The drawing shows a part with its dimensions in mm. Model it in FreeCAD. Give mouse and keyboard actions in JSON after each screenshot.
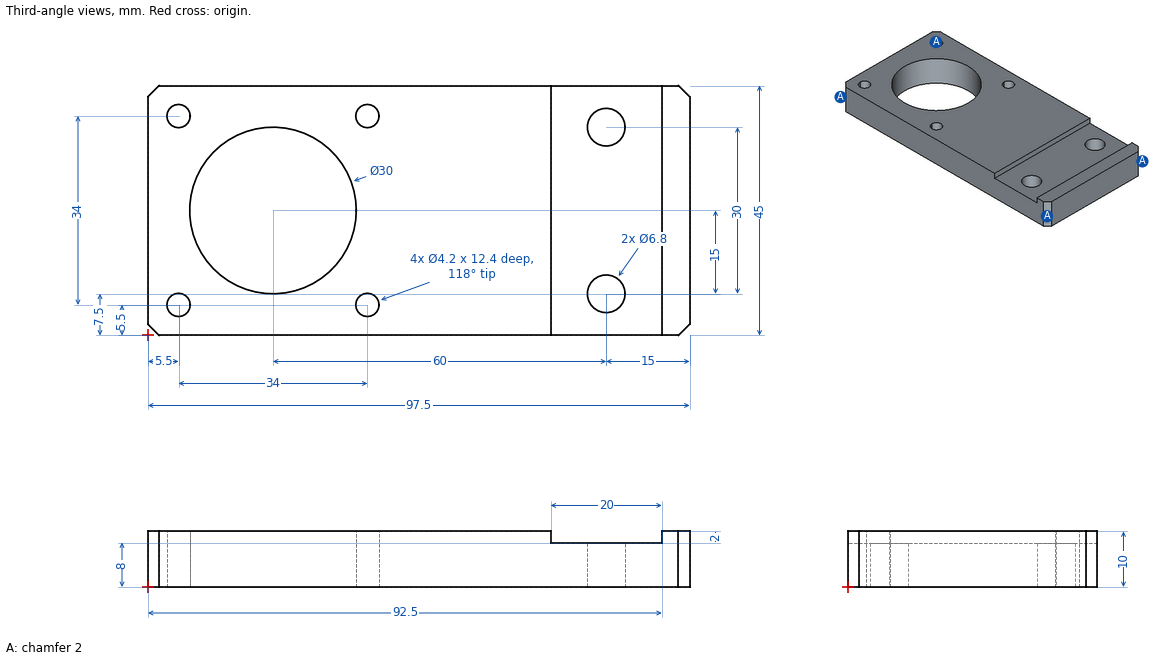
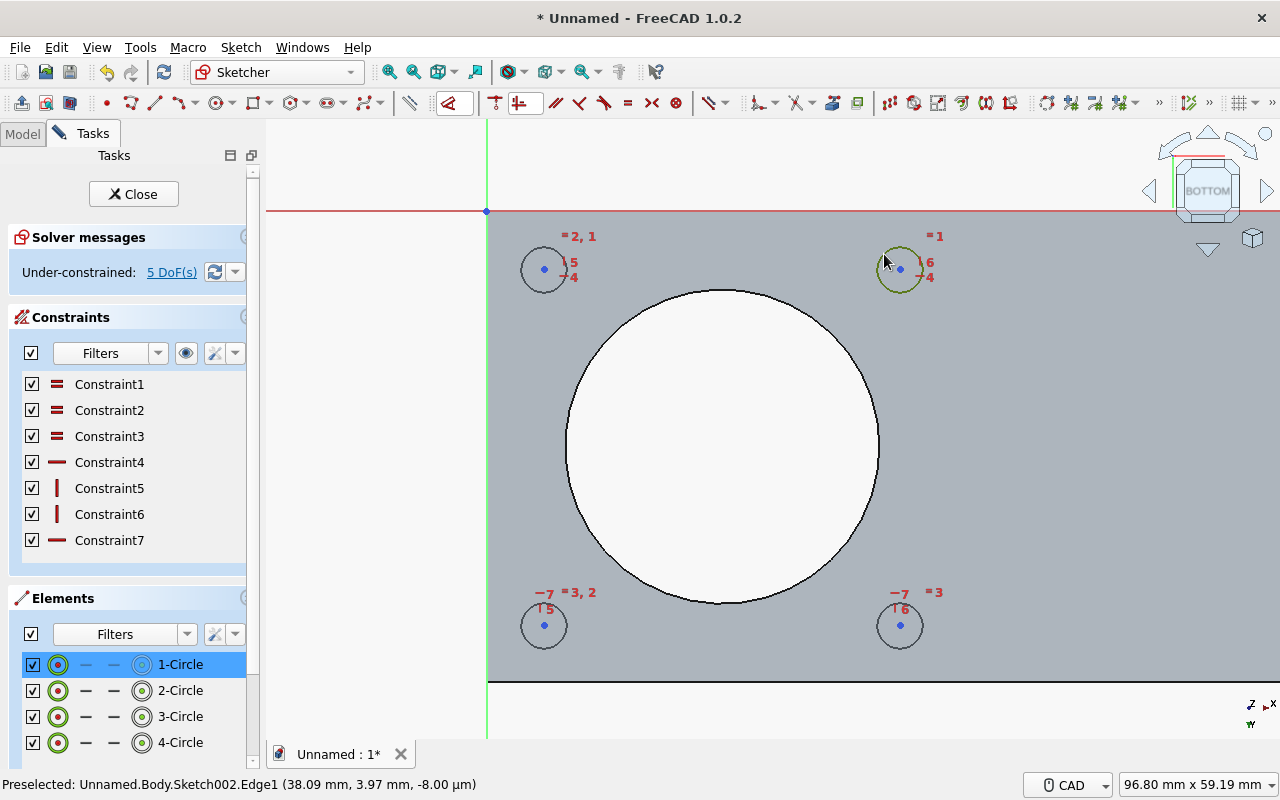
{"action": "left_click", "coordinate": [468, 104]}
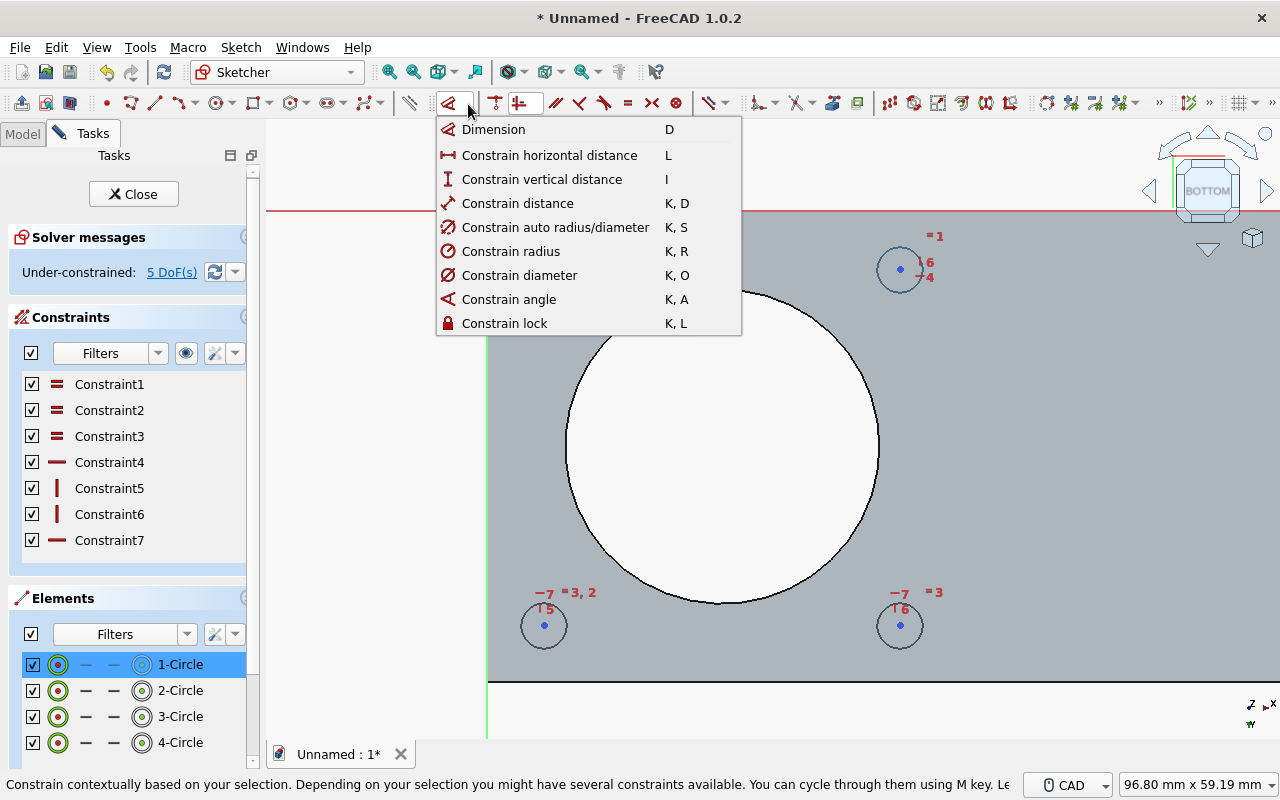
{"action": "left_click", "coordinate": [589, 275]}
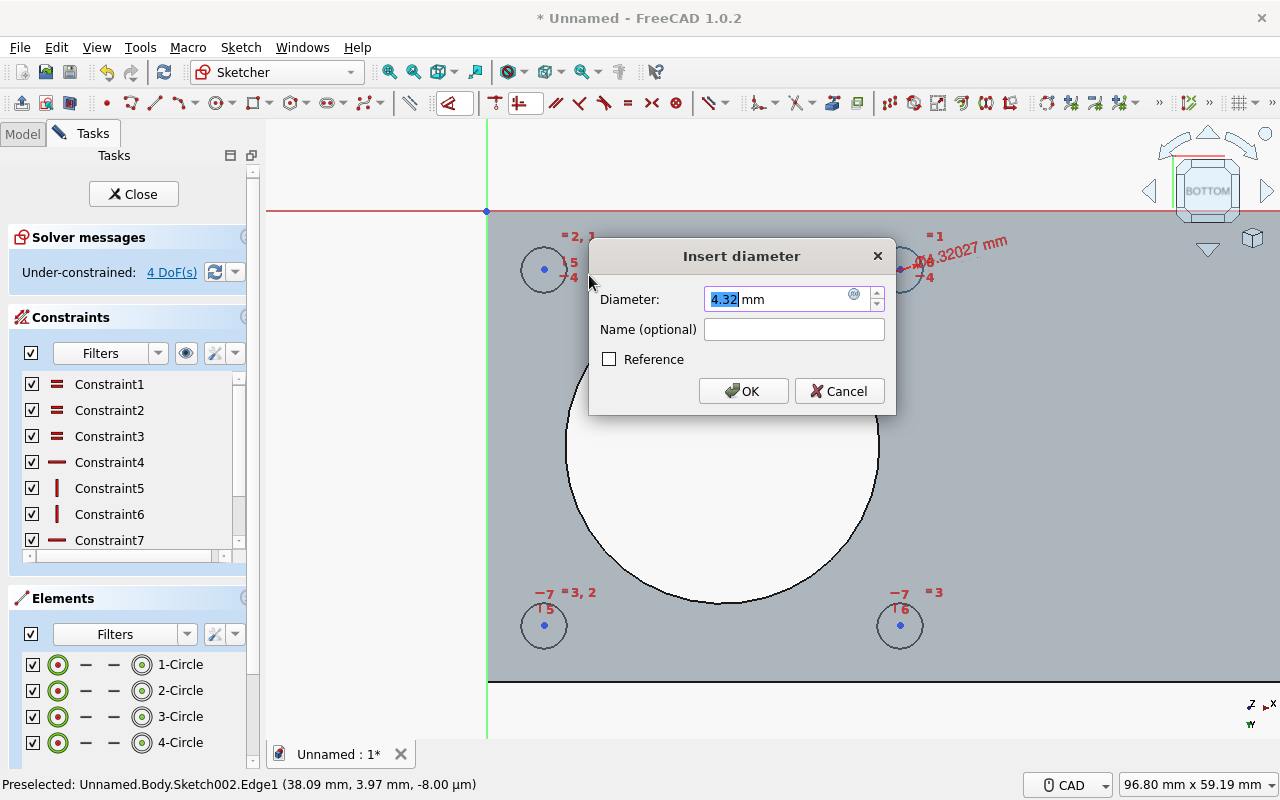
{"action": "type", "text": "4.2"}
{"action": "key", "text": "Return"}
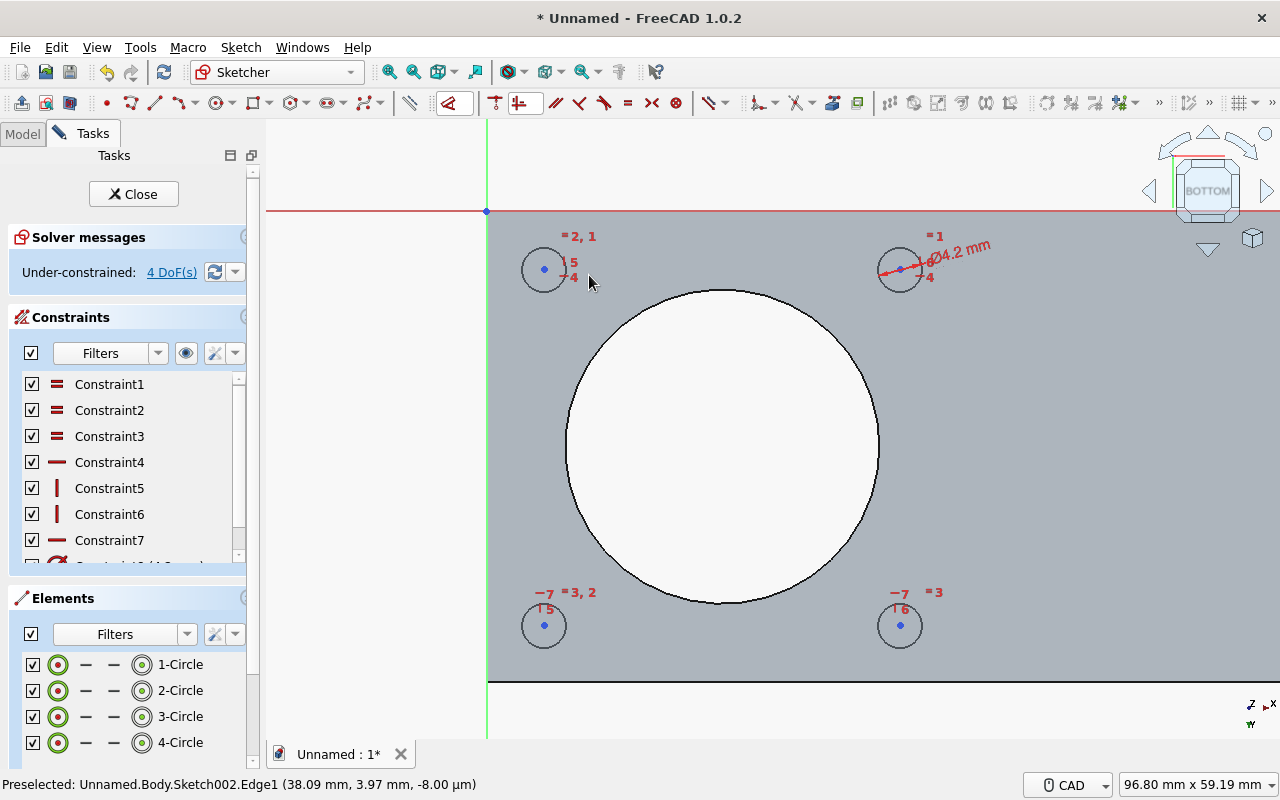
{"action": "left_click", "coordinate": [900, 270]}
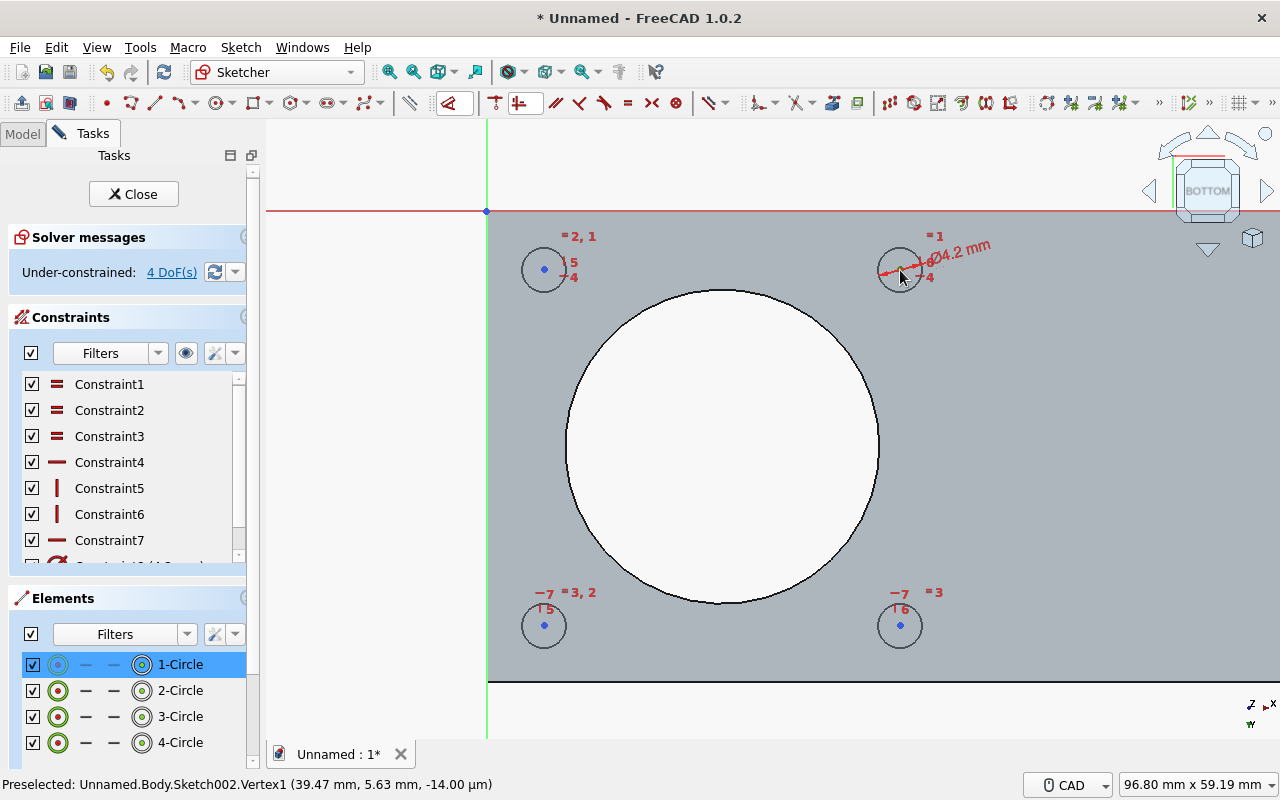
{"action": "key", "text": "i"}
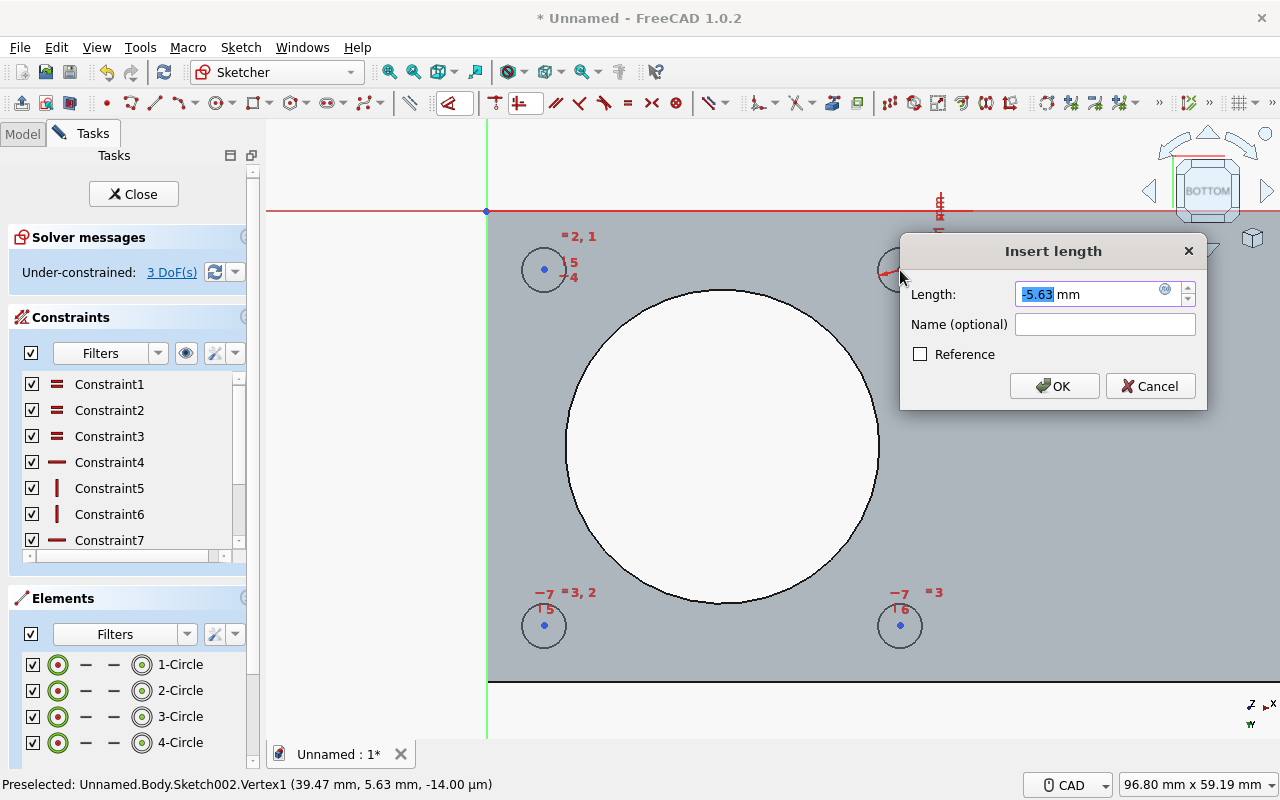
{"action": "type", "text": "-5.5"}
{"action": "key", "text": "Return"}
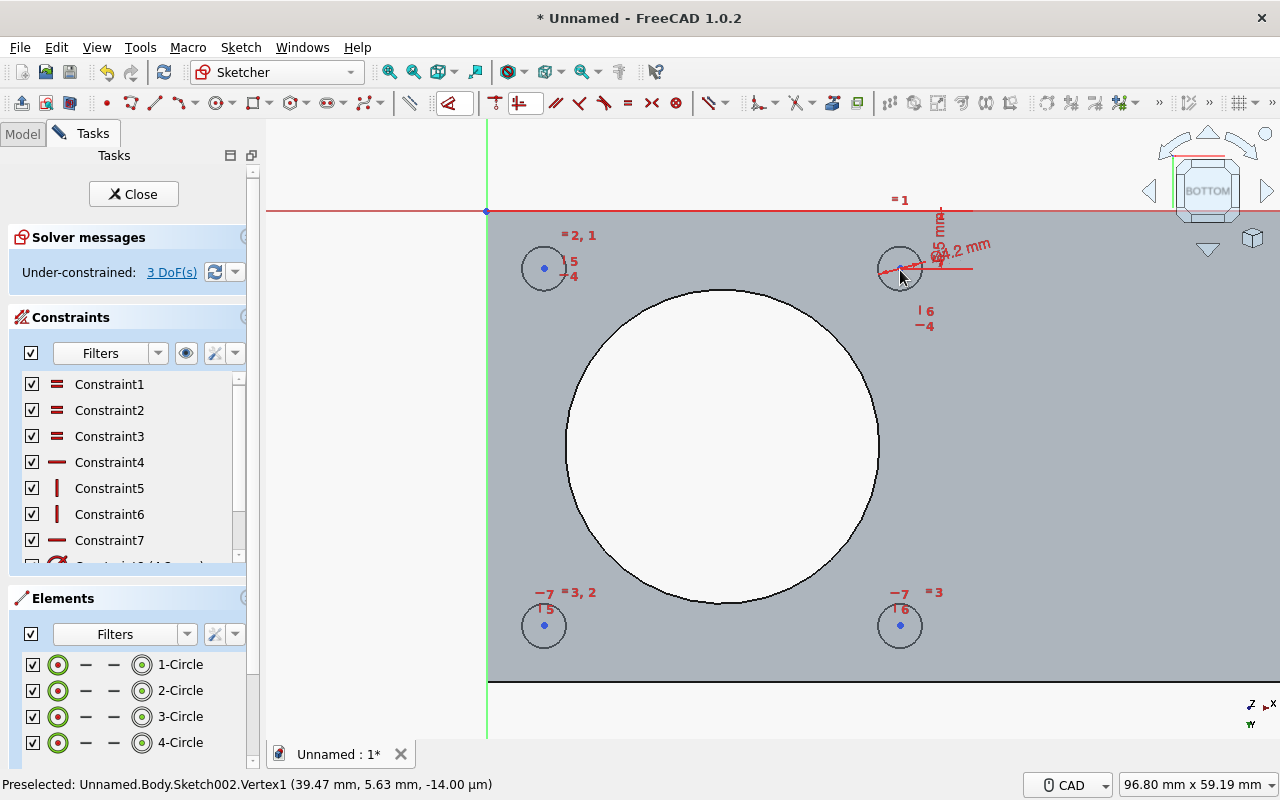
{"action": "left_click", "coordinate": [544, 269]}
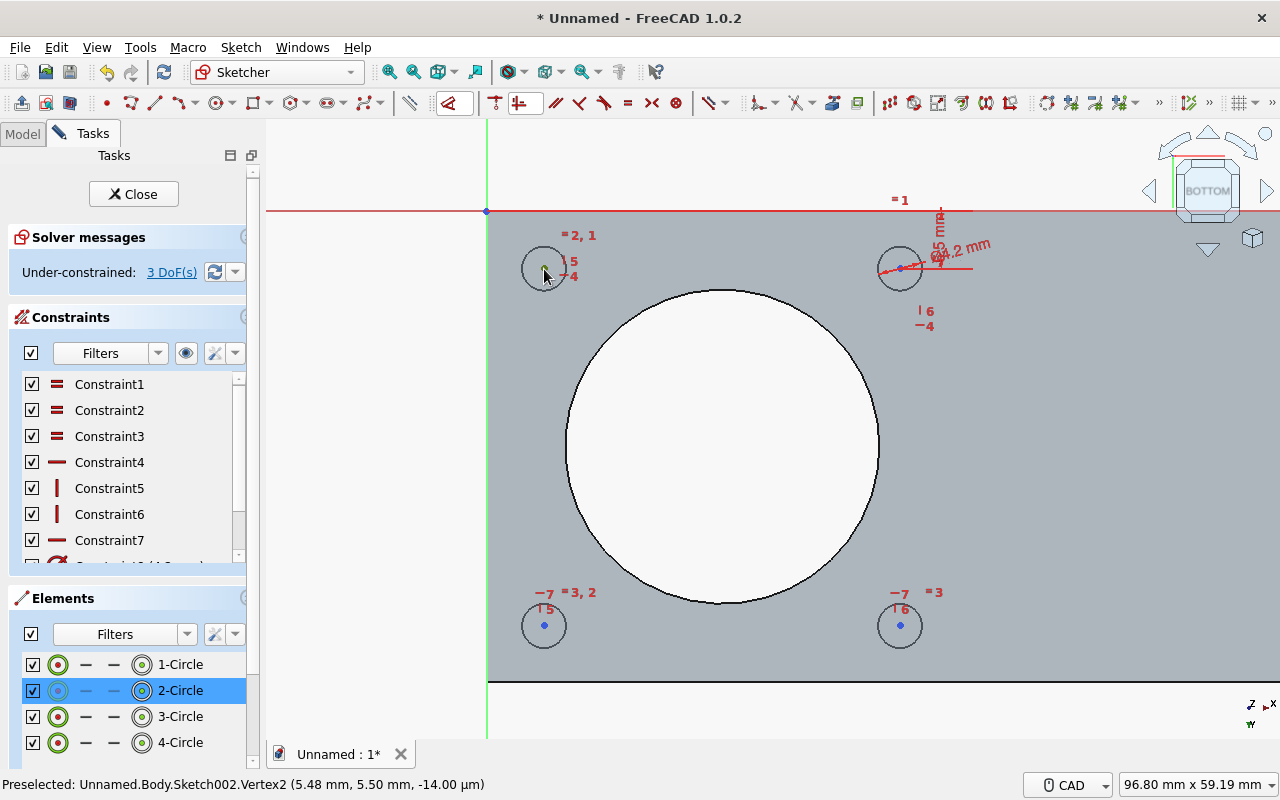
{"action": "key", "text": "l"}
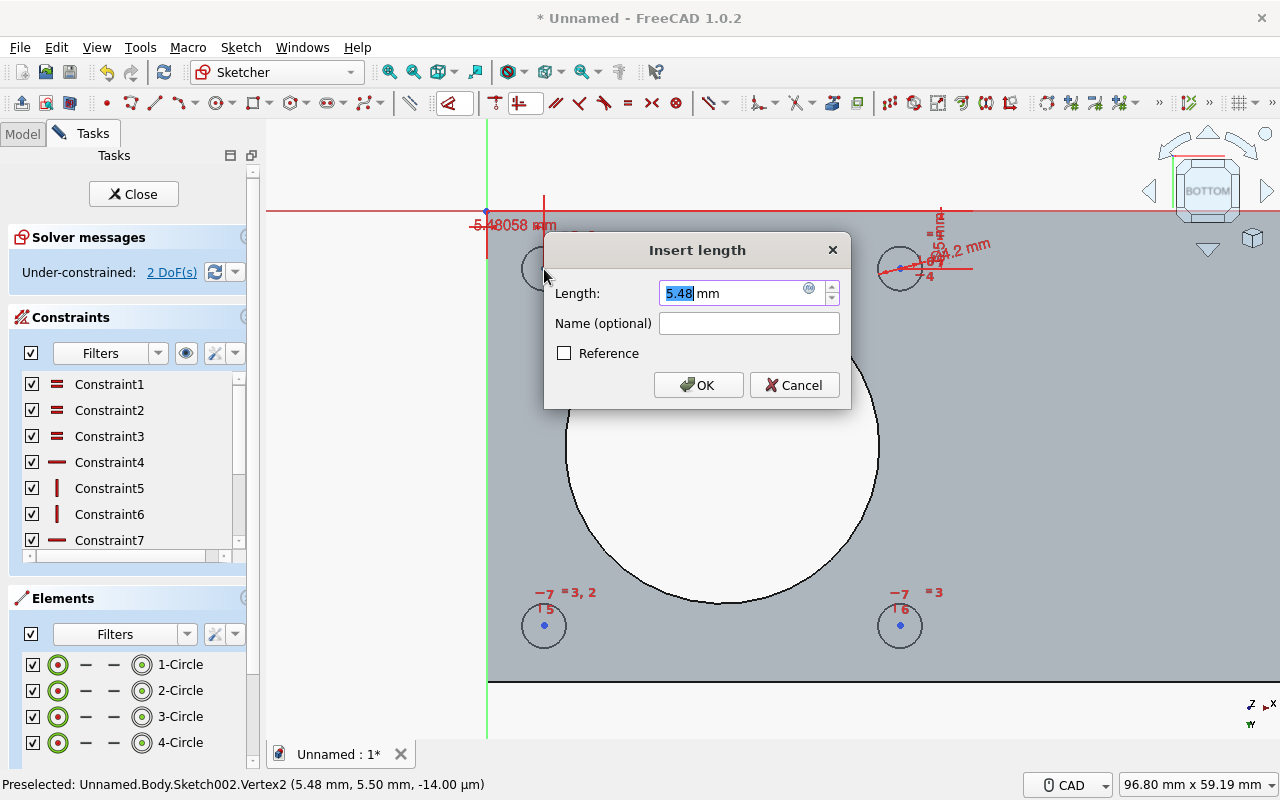
{"action": "type", "text": "5.5"}
{"action": "key", "text": "Return"}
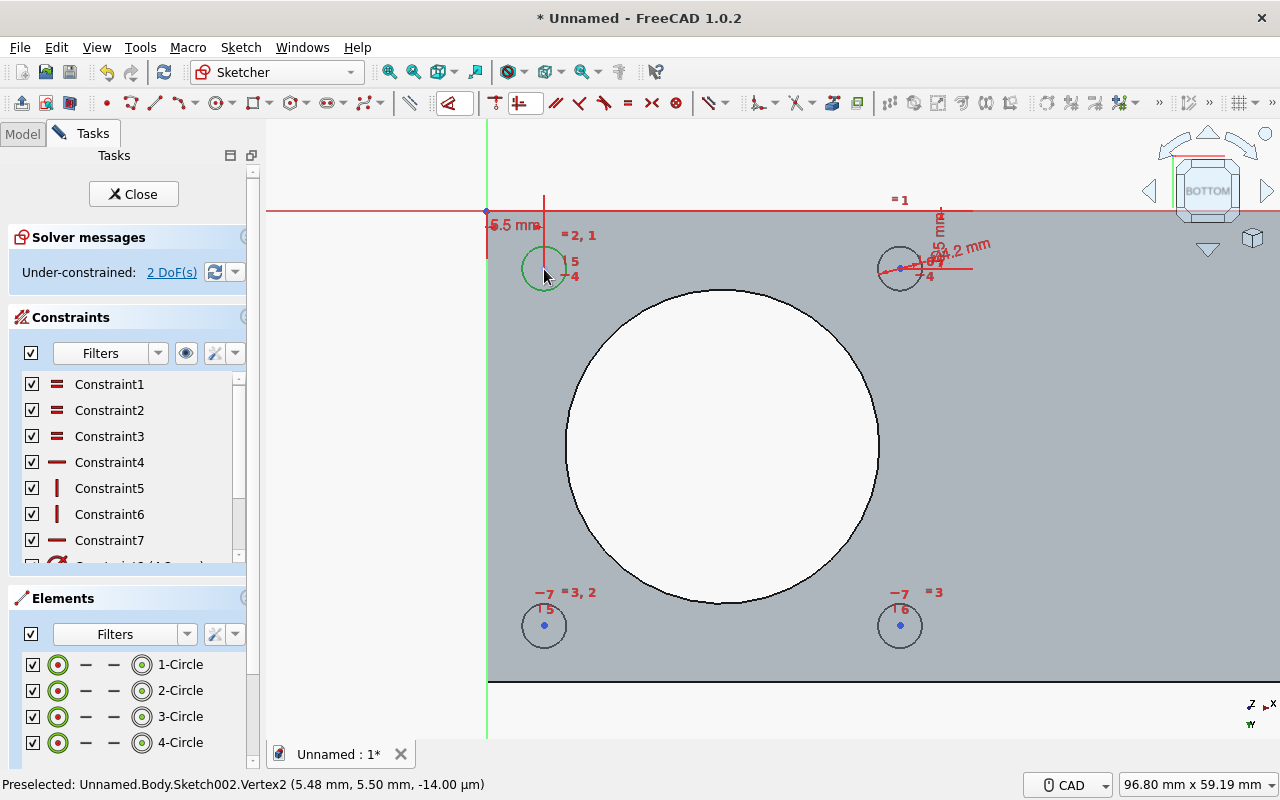
{"action": "left_click", "coordinate": [900, 269]}